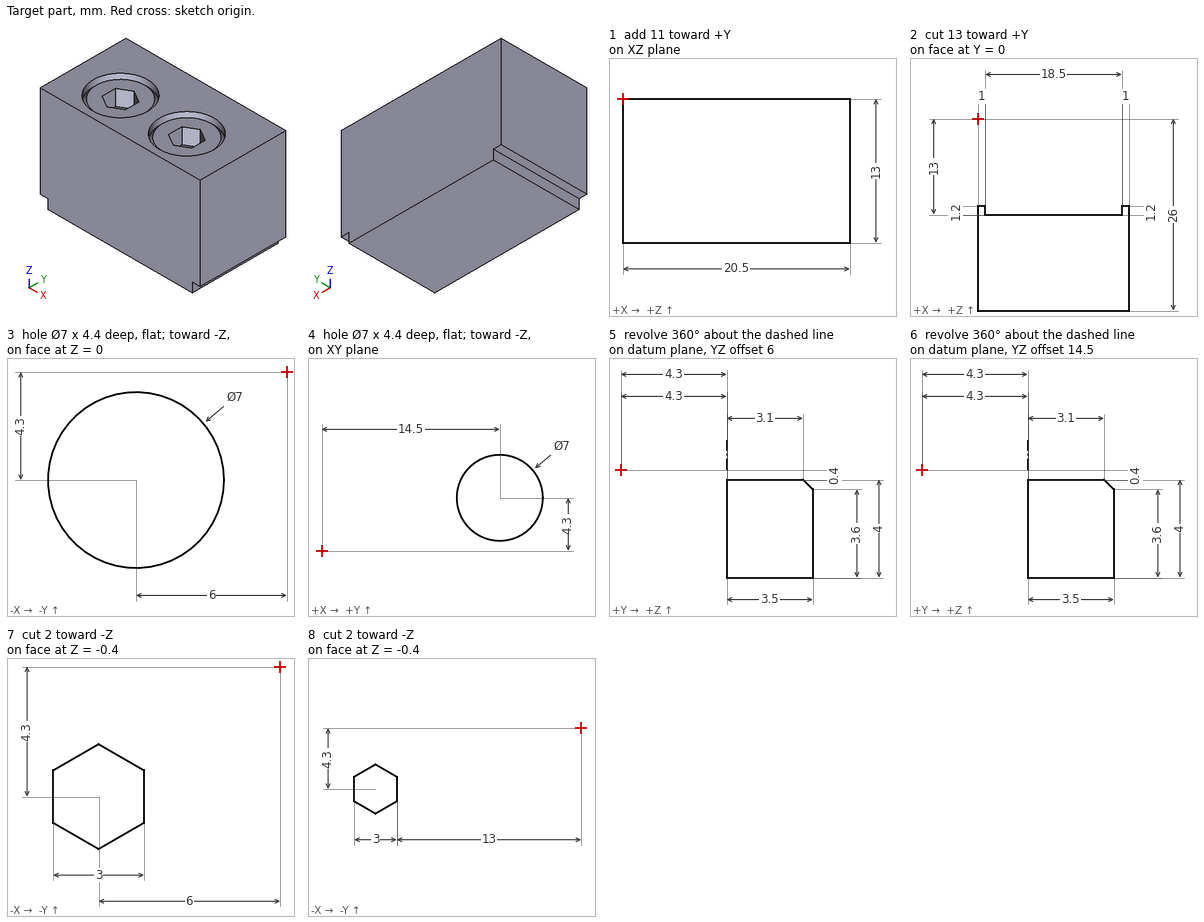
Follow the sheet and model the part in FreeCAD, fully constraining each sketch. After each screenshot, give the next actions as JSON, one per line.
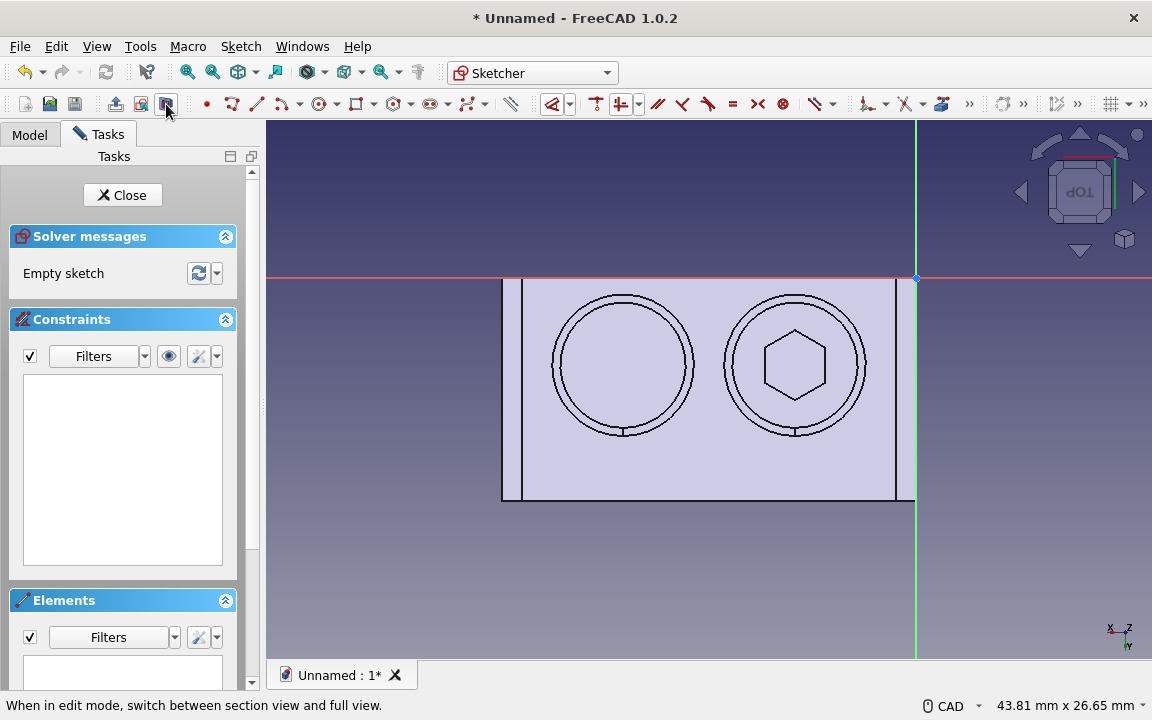
{"action": "scroll", "coordinate": [619, 359], "scroll_direction": "up", "scroll_amount": 8}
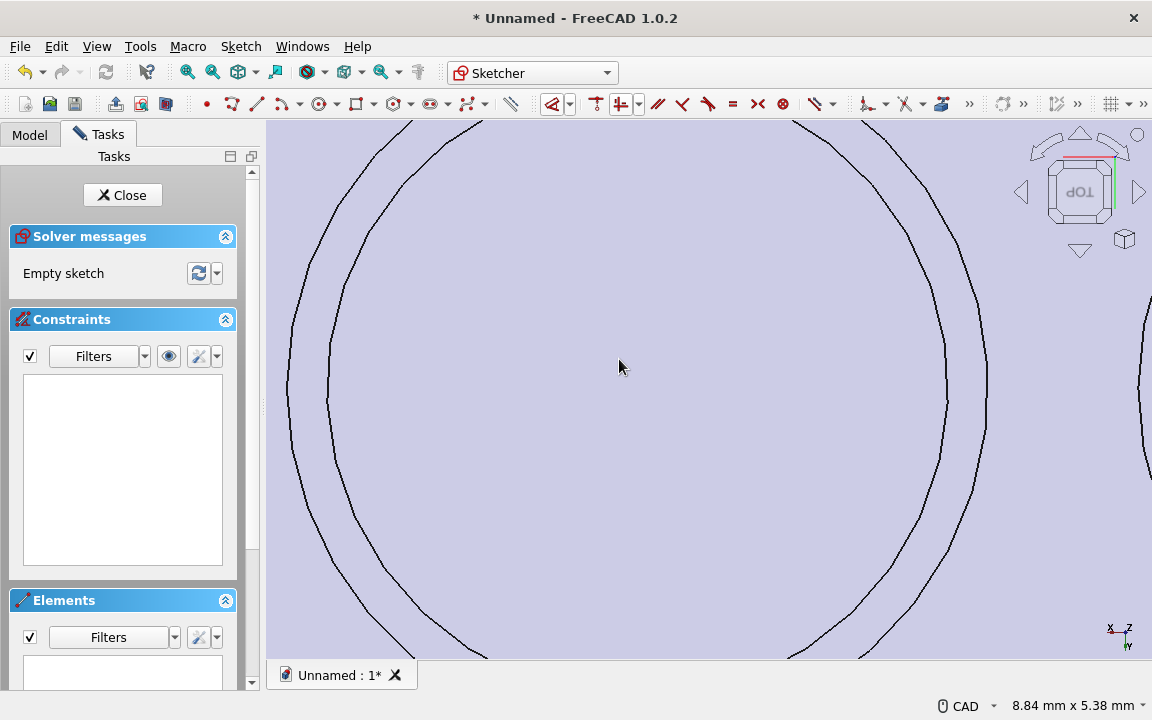
{"action": "left_click", "coordinate": [392, 104]}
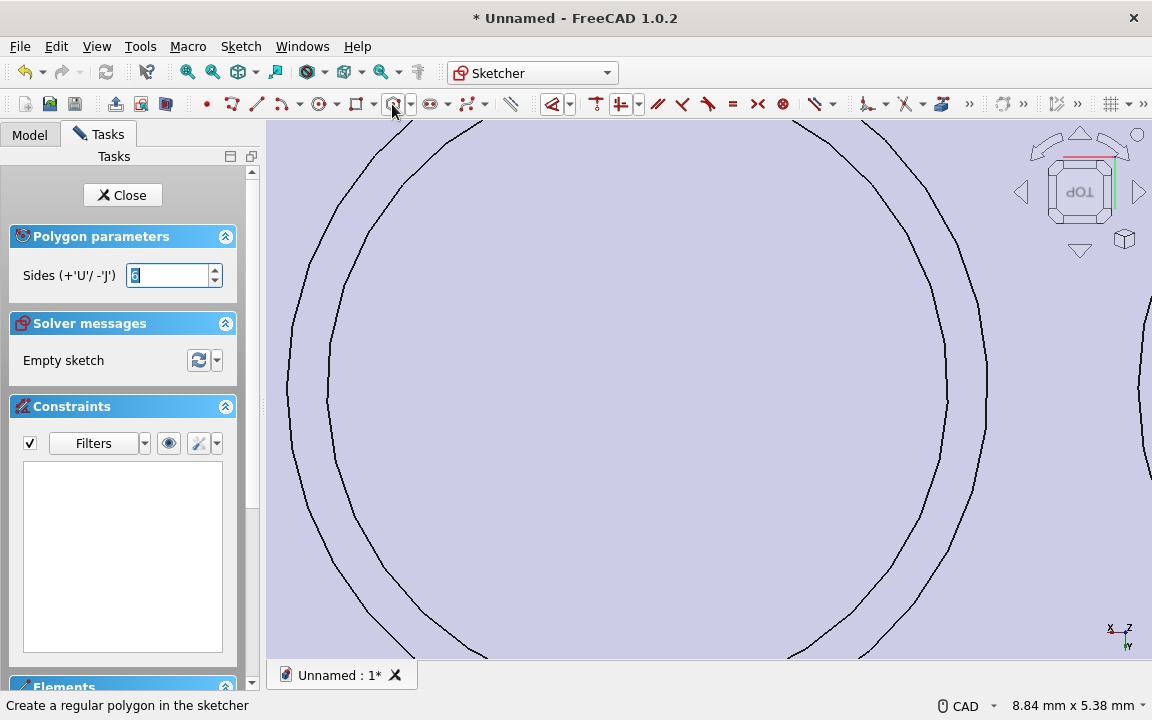
{"action": "left_click", "coordinate": [637, 388]}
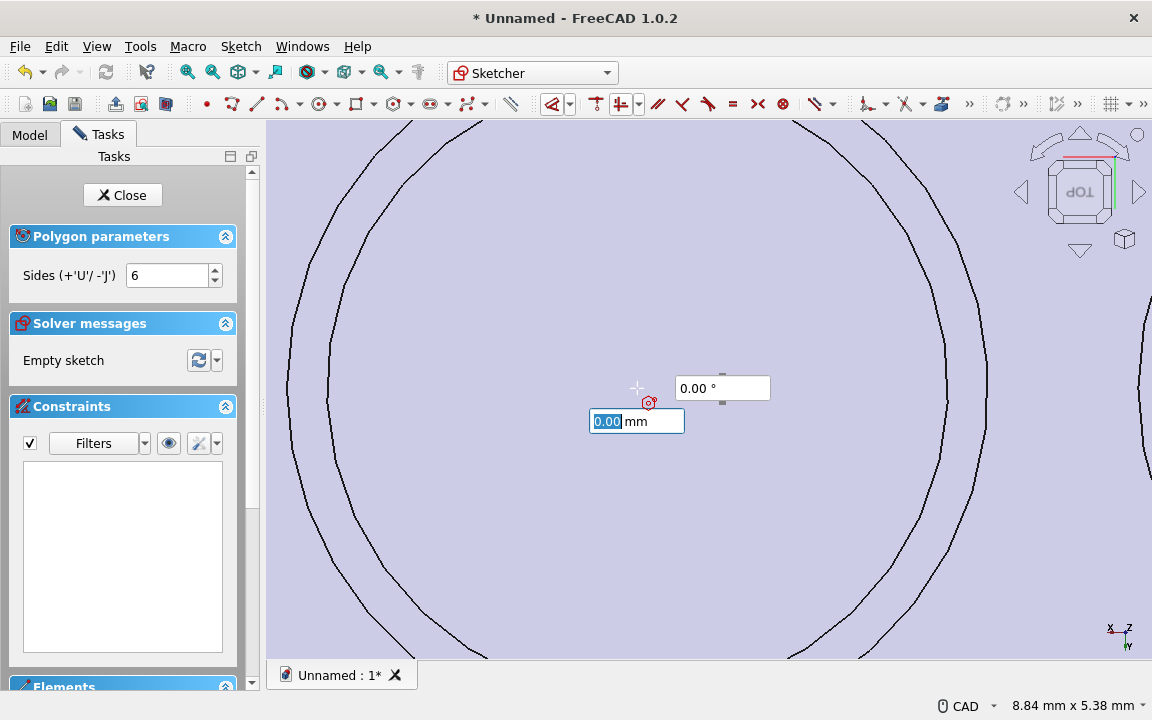
{"action": "left_click", "coordinate": [637, 562]}
{"action": "right_click", "coordinate": [637, 562]}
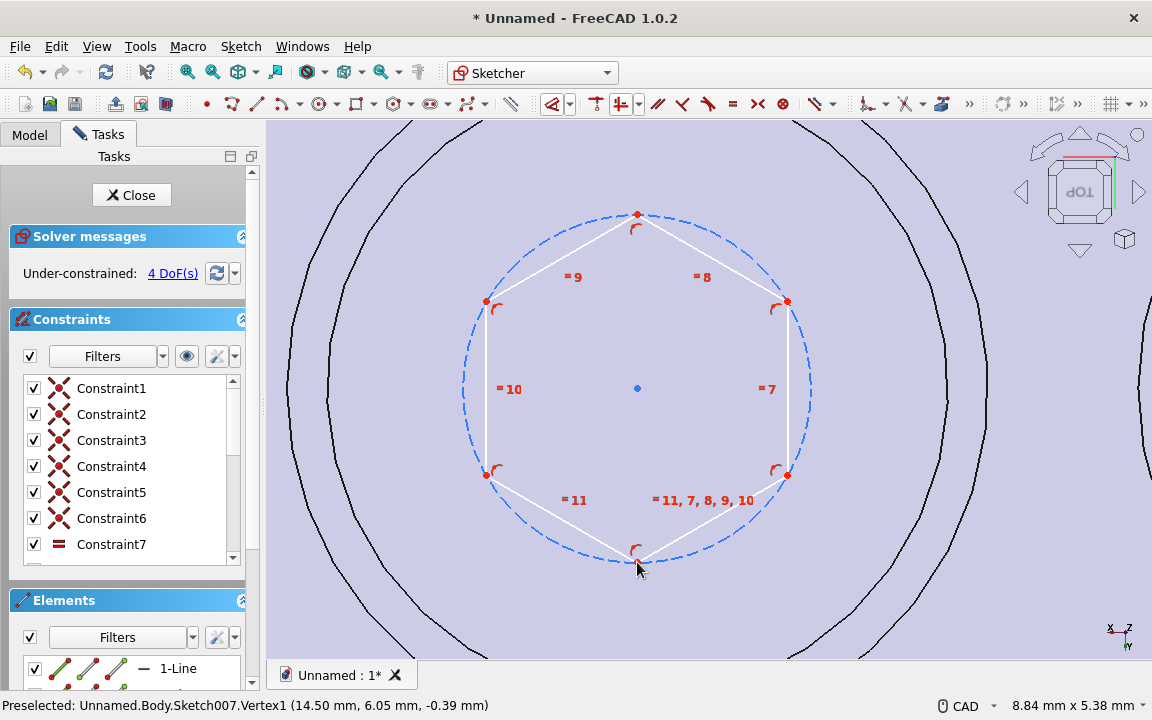
{"action": "left_click", "coordinate": [788, 424]}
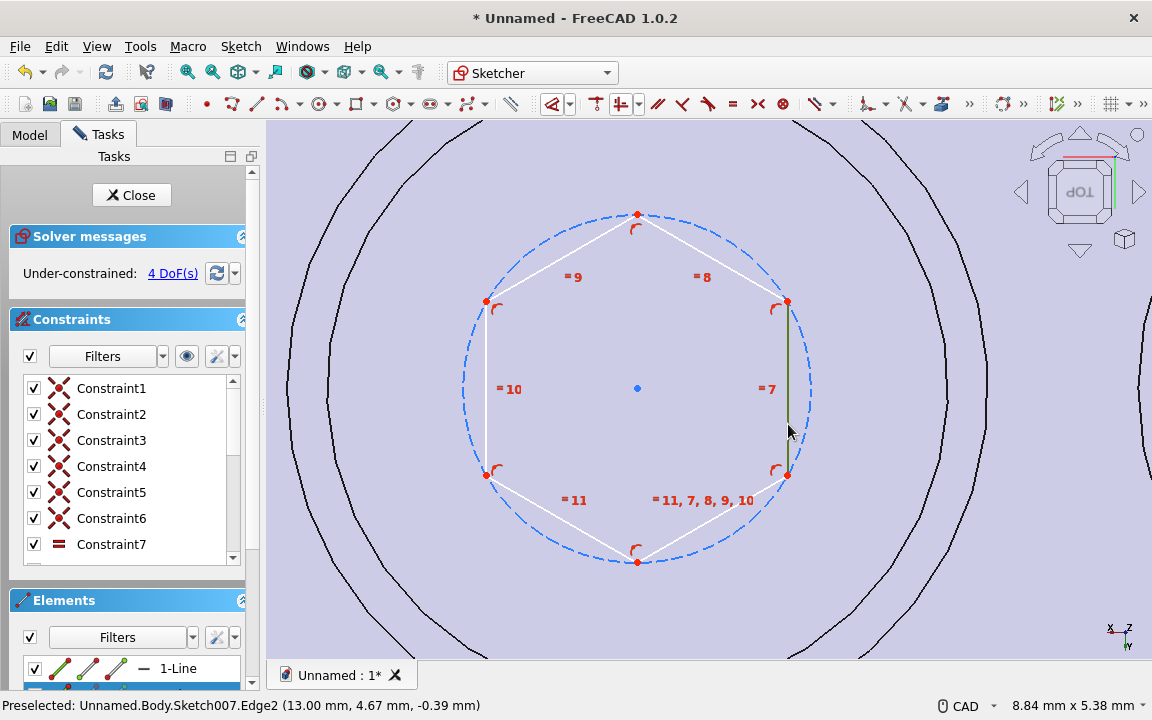
{"action": "key", "text": "v"}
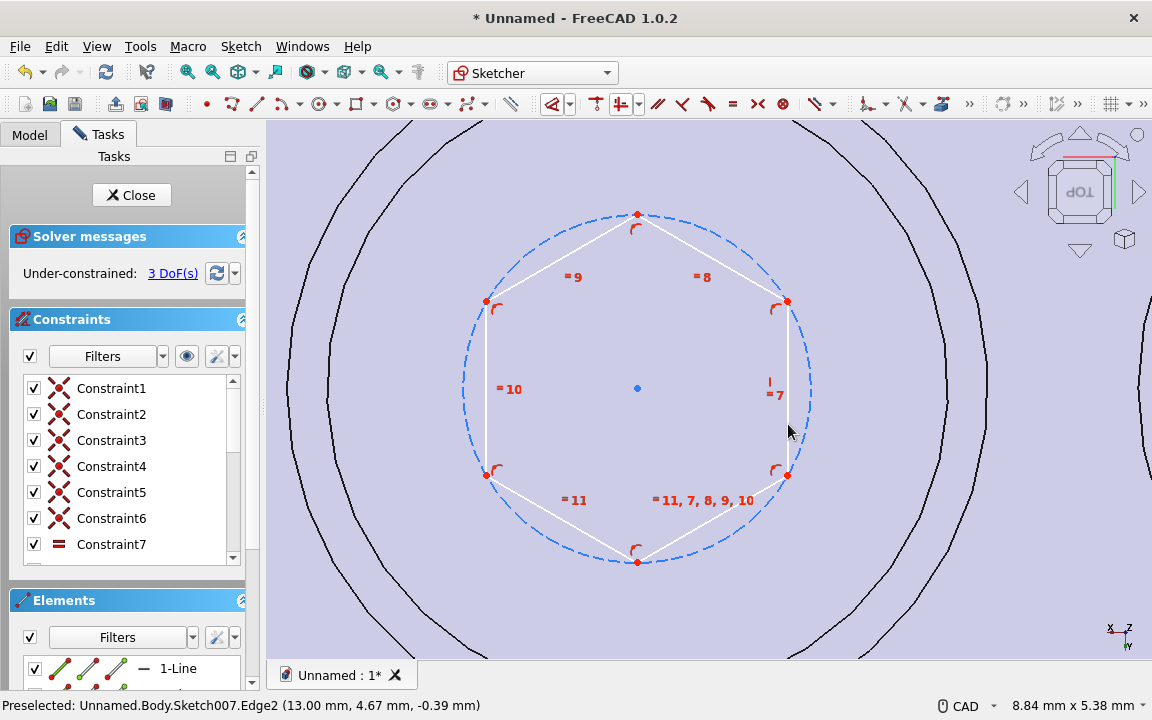
{"action": "left_click", "coordinate": [486, 302]}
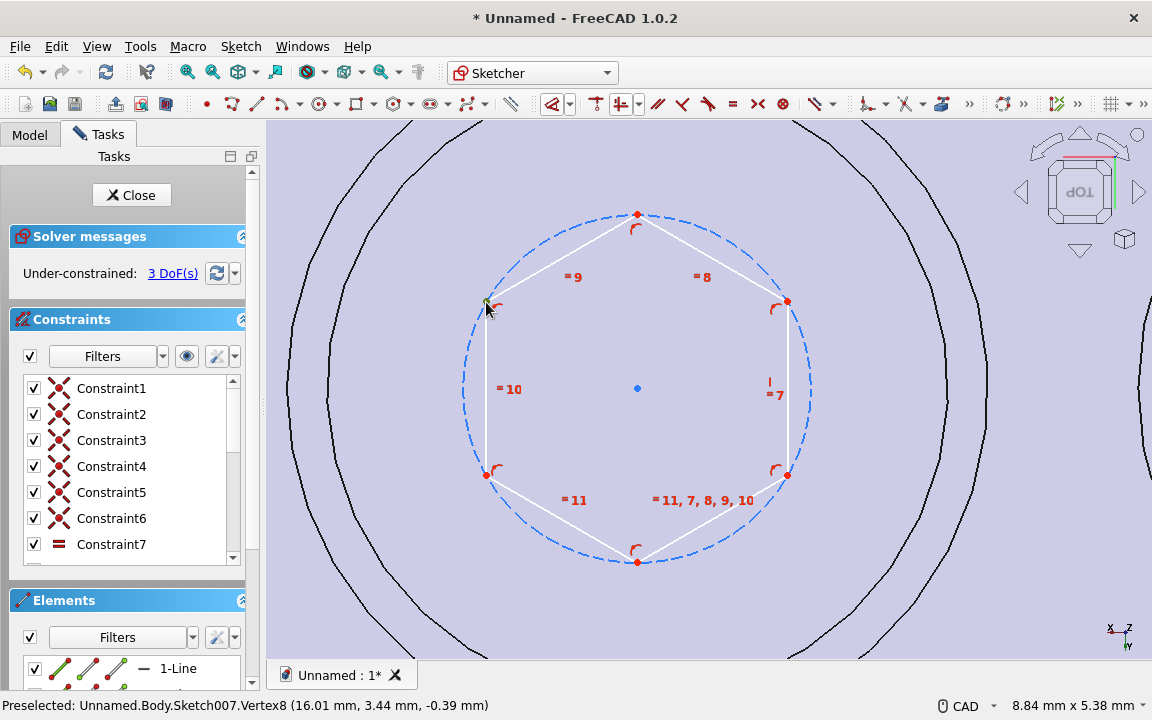
{"action": "left_click", "coordinate": [788, 476]}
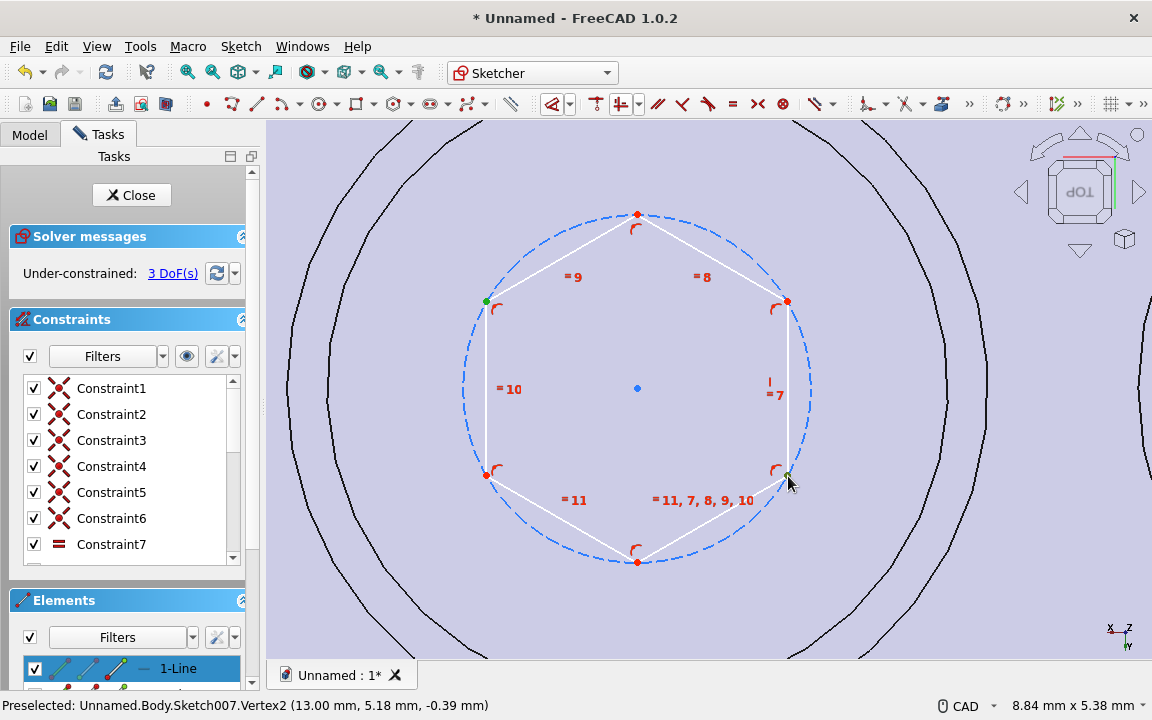
{"action": "left_click", "coordinate": [570, 104]}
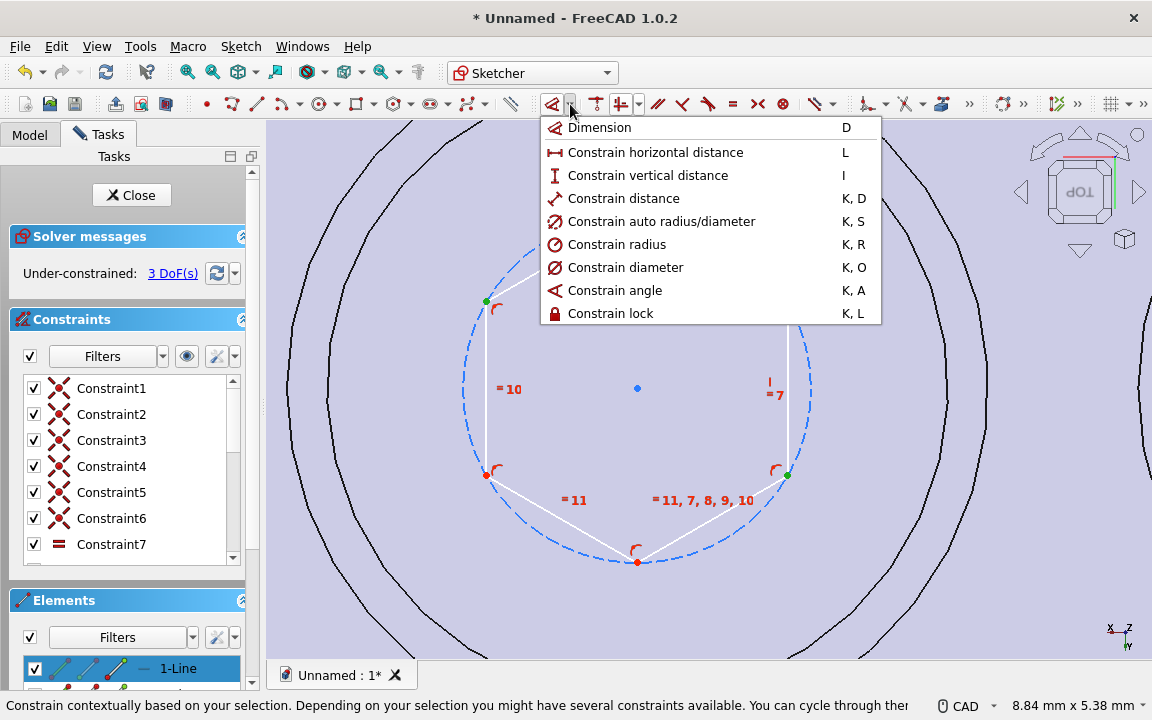
{"action": "left_click", "coordinate": [711, 152]}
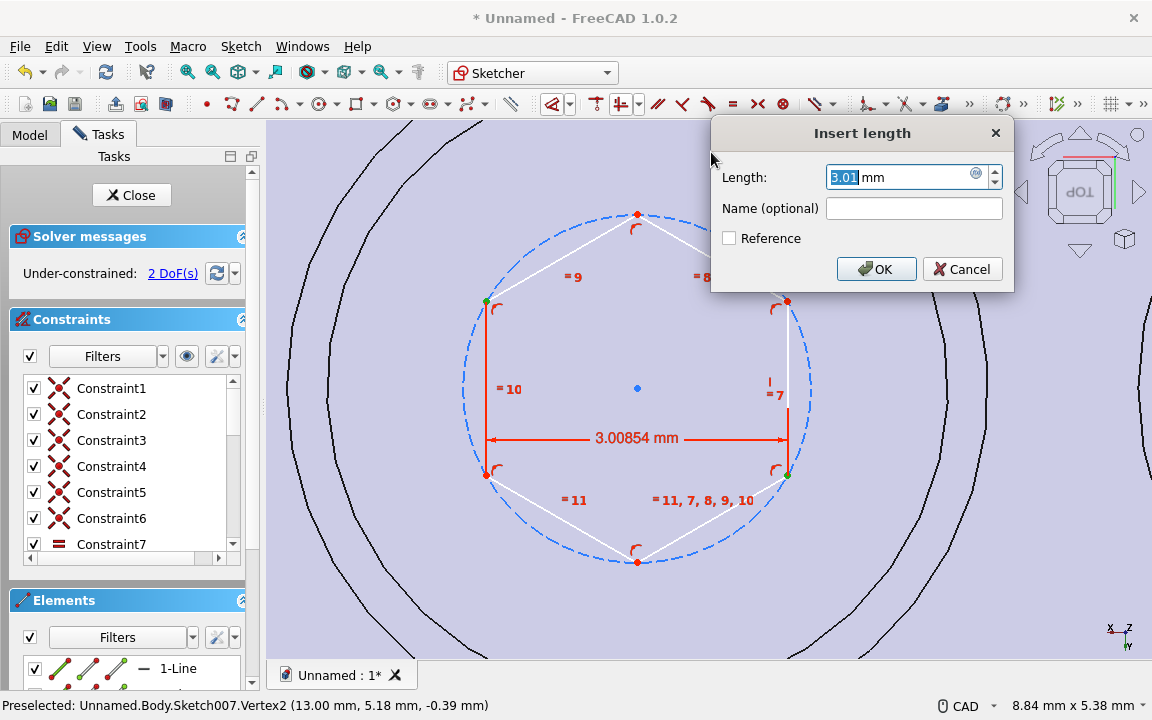
{"action": "type", "text": "3"}
{"action": "key", "text": "Return"}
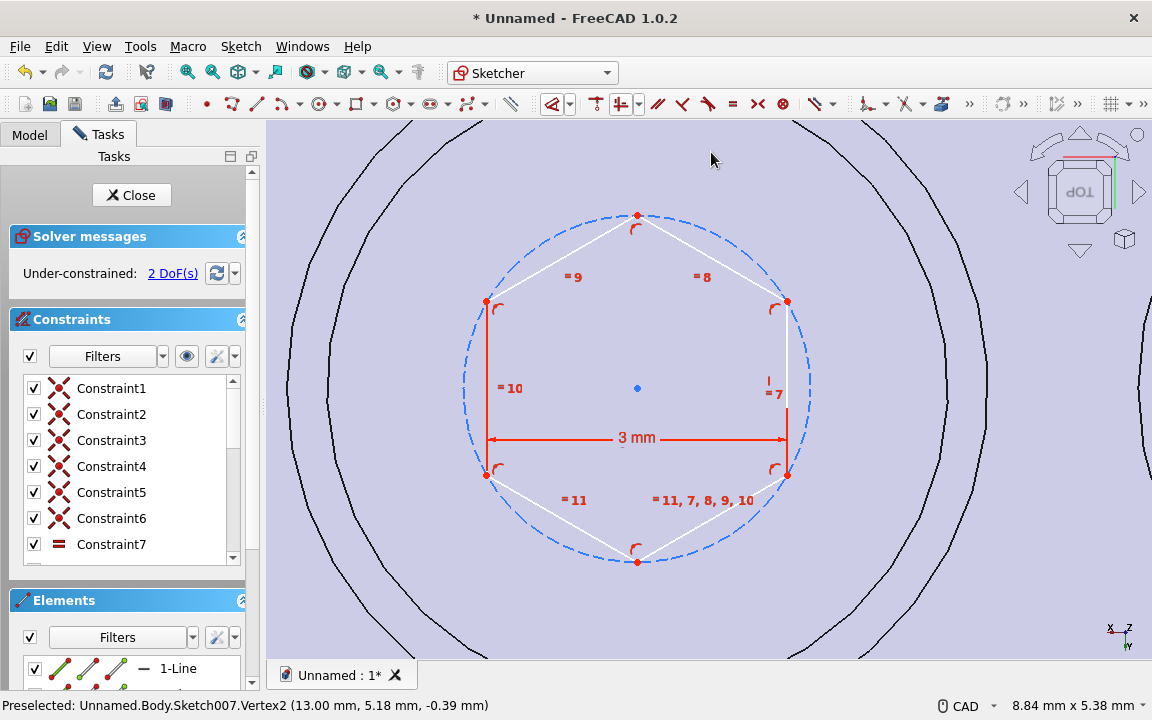
{"action": "left_click", "coordinate": [787, 476]}